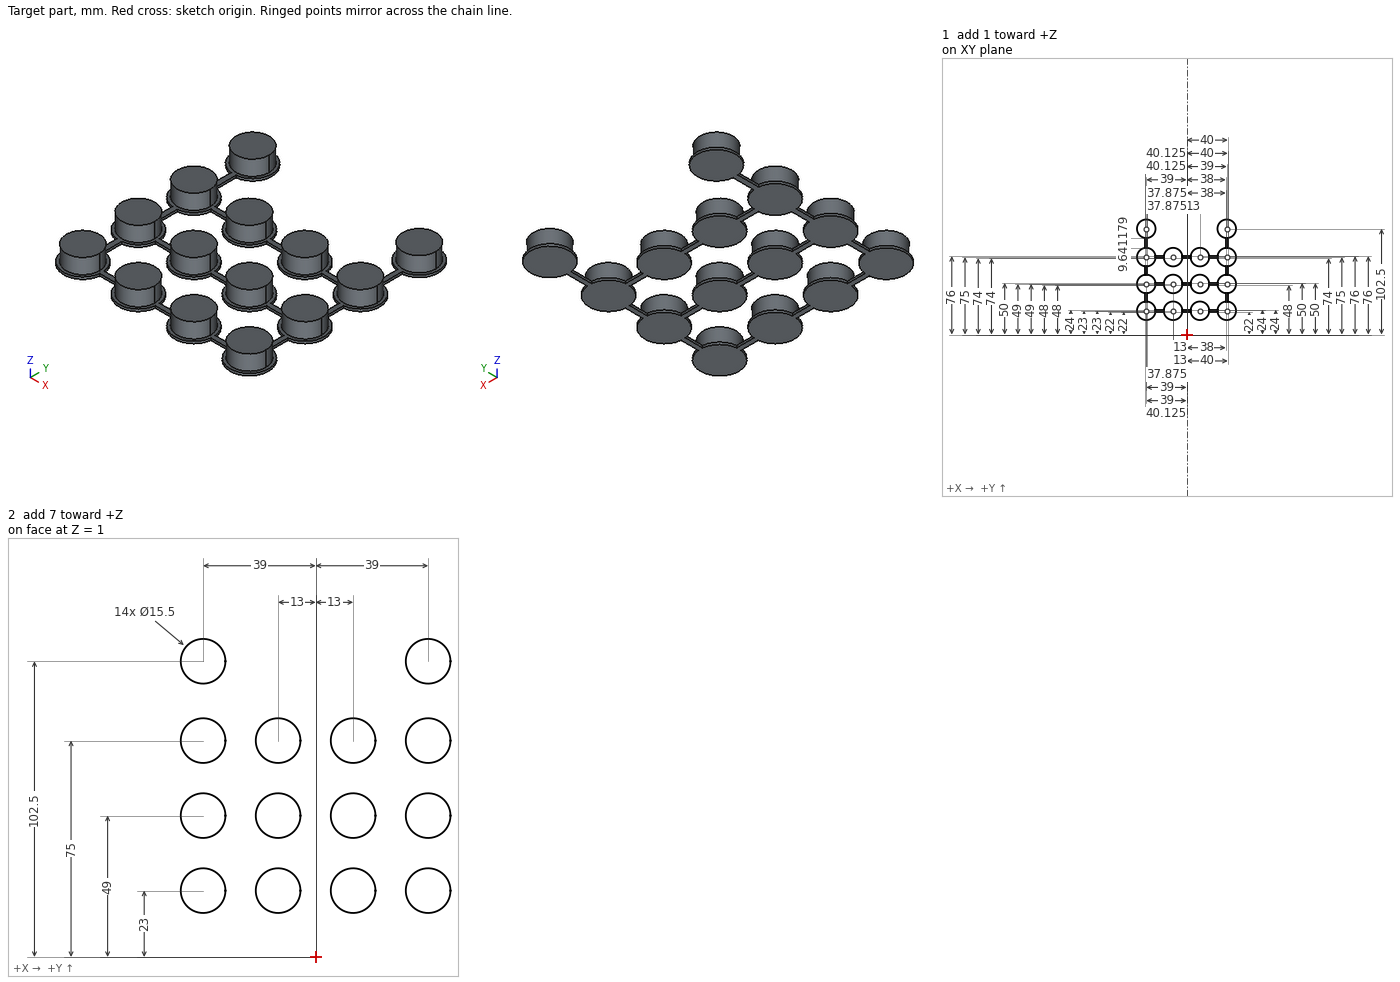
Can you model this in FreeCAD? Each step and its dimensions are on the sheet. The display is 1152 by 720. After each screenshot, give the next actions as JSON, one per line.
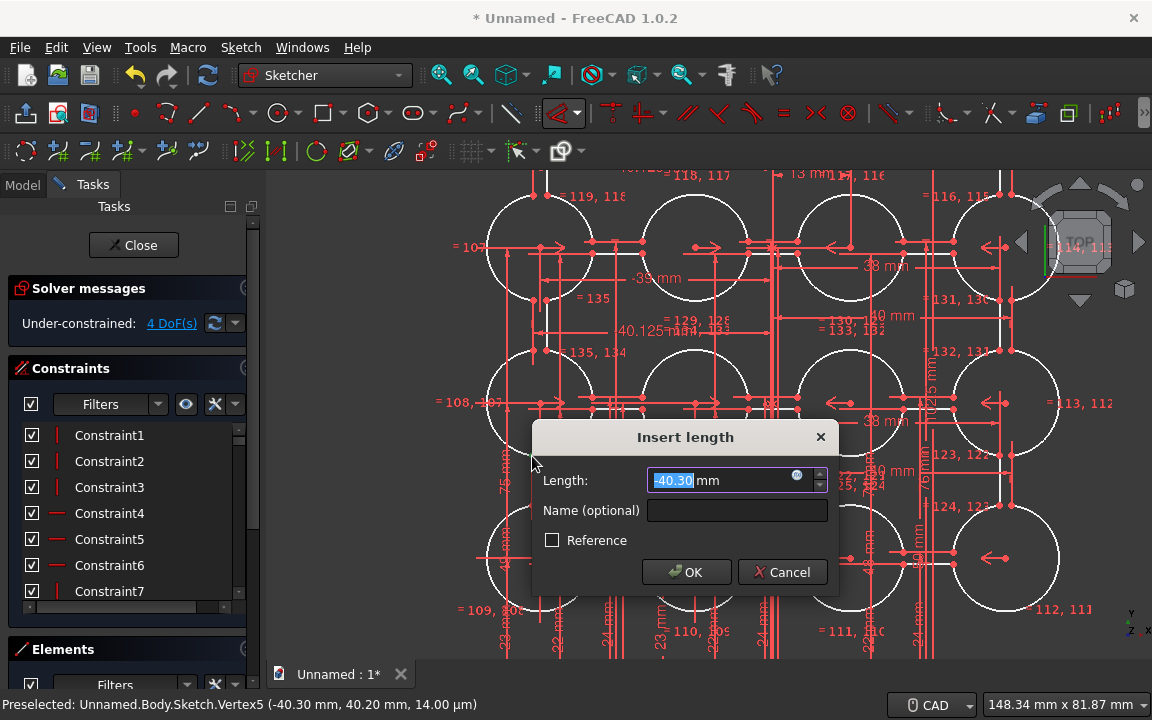
{"action": "type", "text": "-40.125"}
{"action": "key", "text": "Return"}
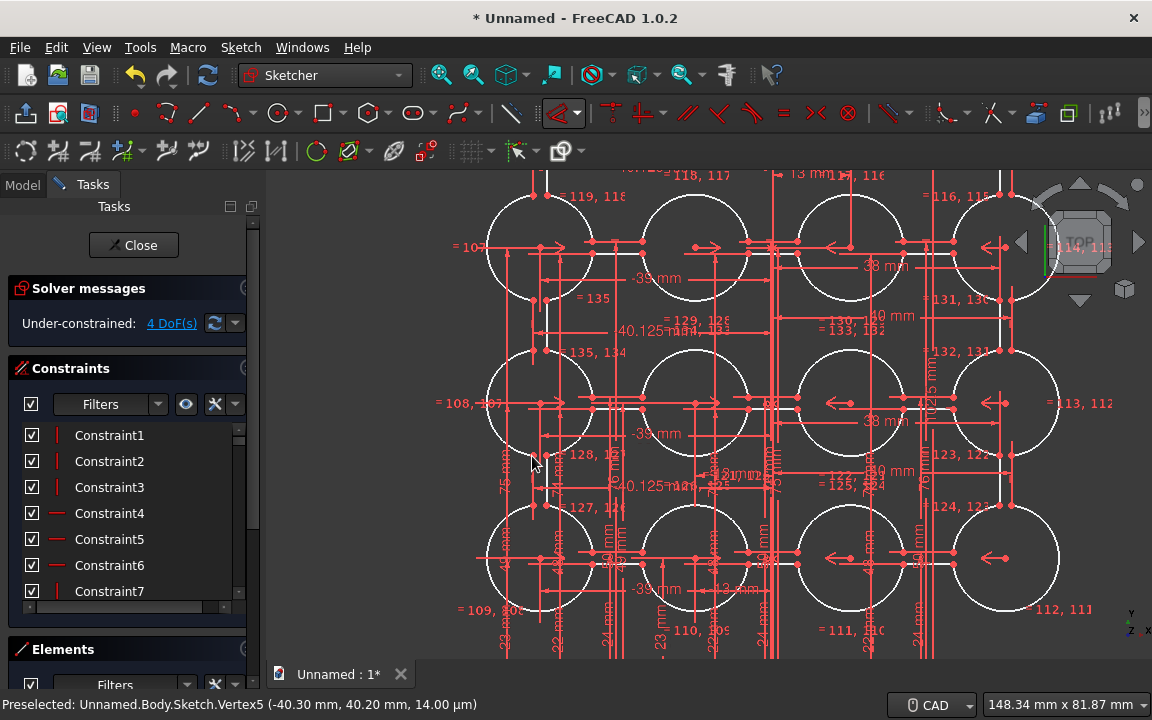
{"action": "scroll", "coordinate": [532, 457], "scroll_direction": "down", "scroll_amount": 4}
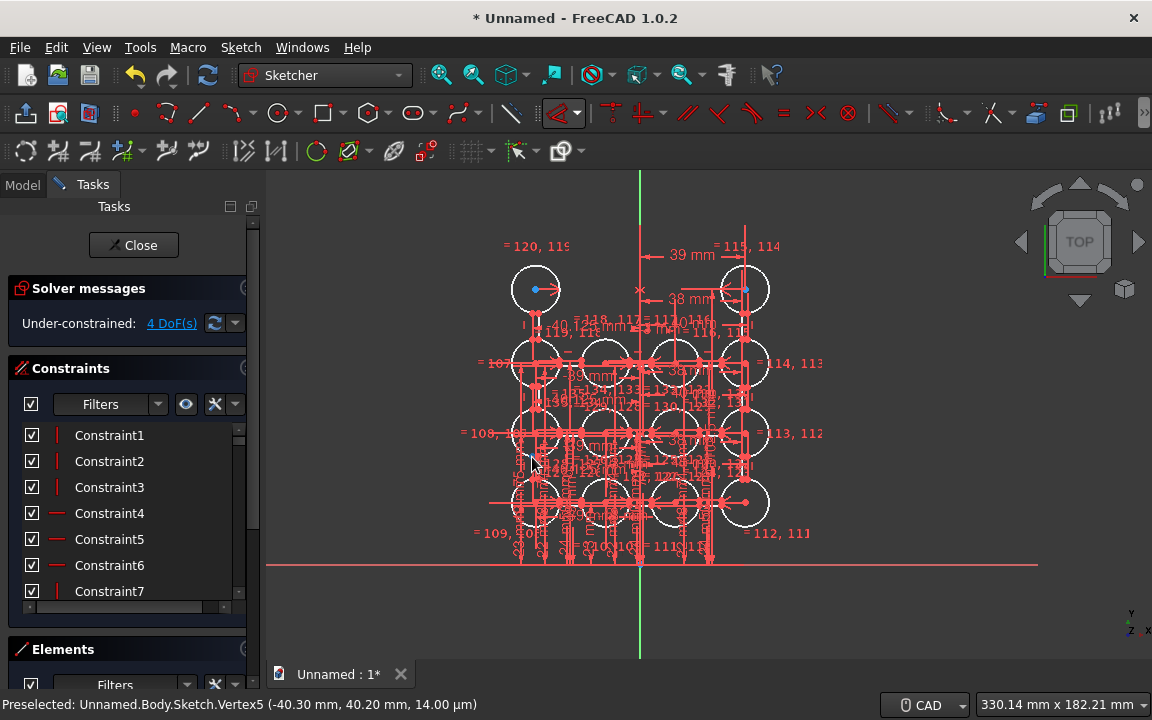
{"action": "scroll", "coordinate": [539, 340], "scroll_direction": "up", "scroll_amount": 4}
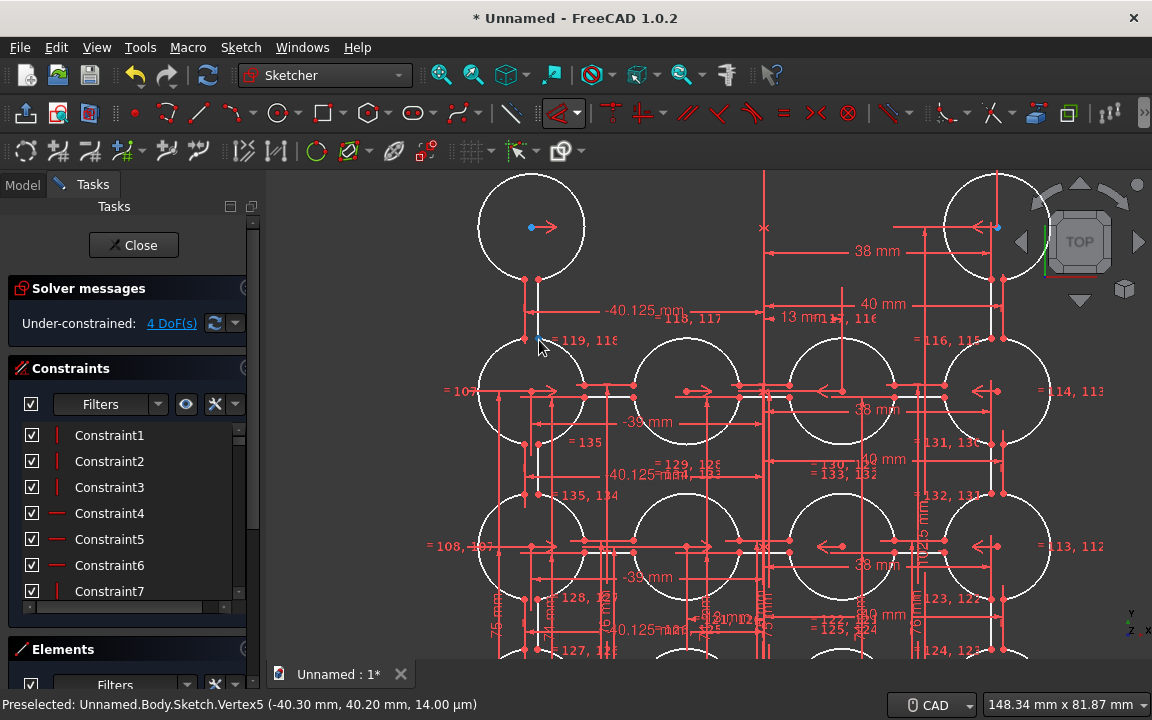
{"action": "left_click", "coordinate": [538, 339]}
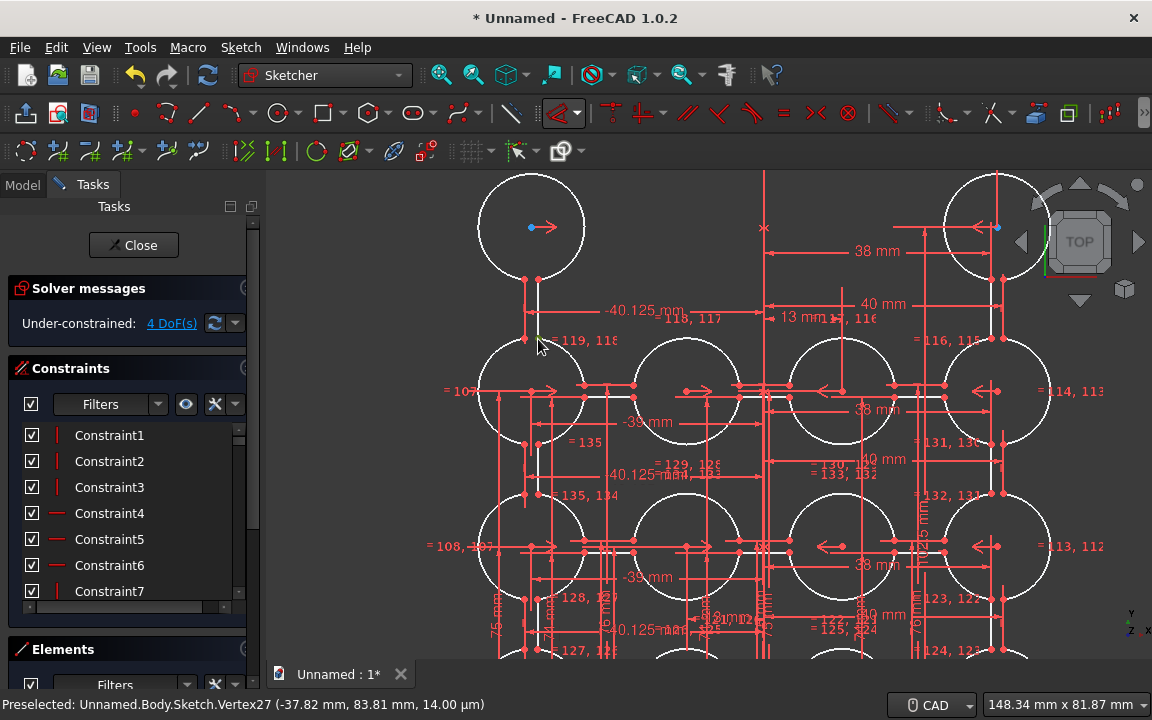
{"action": "left_click", "coordinate": [580, 114]}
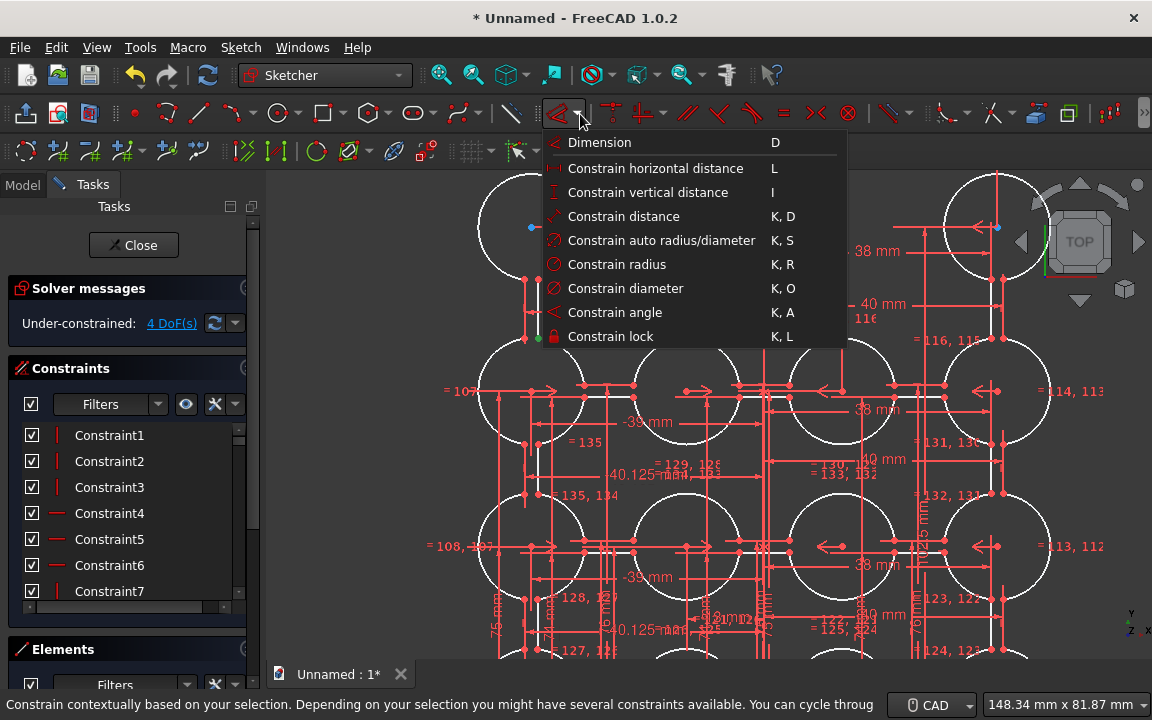
{"action": "left_click", "coordinate": [695, 168]}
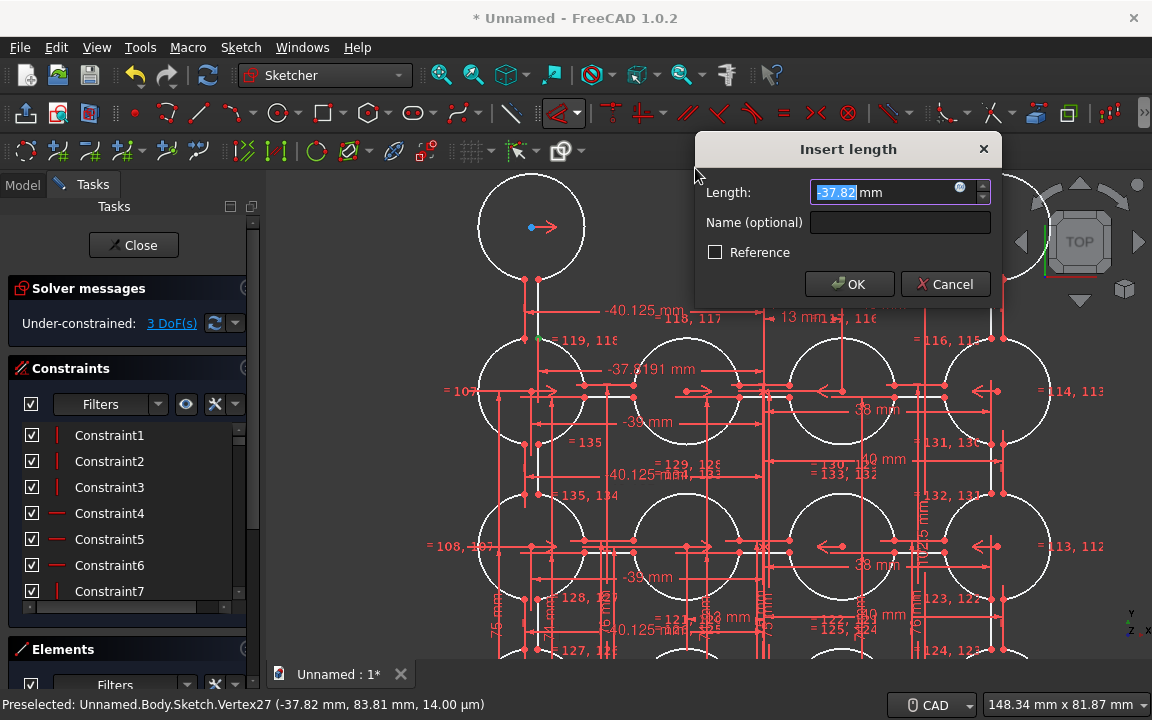
{"action": "type", "text": "-37.875"}
{"action": "key", "text": "Return"}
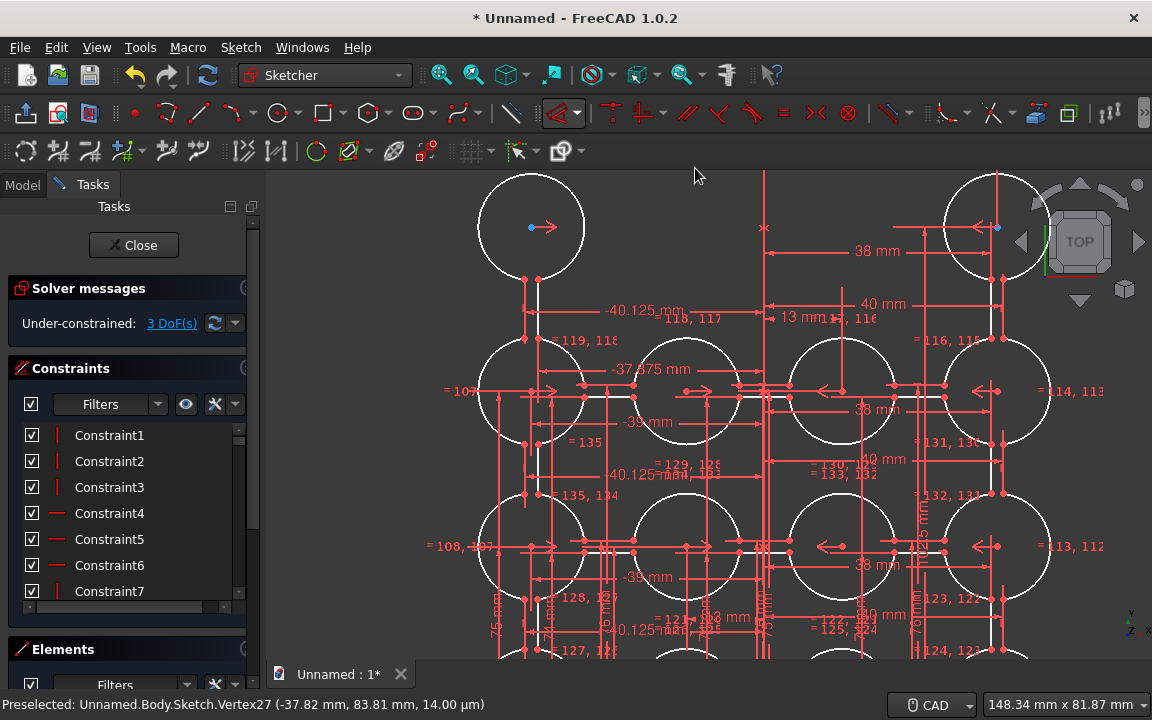
{"action": "scroll", "coordinate": [539, 340], "scroll_direction": "down", "scroll_amount": 4}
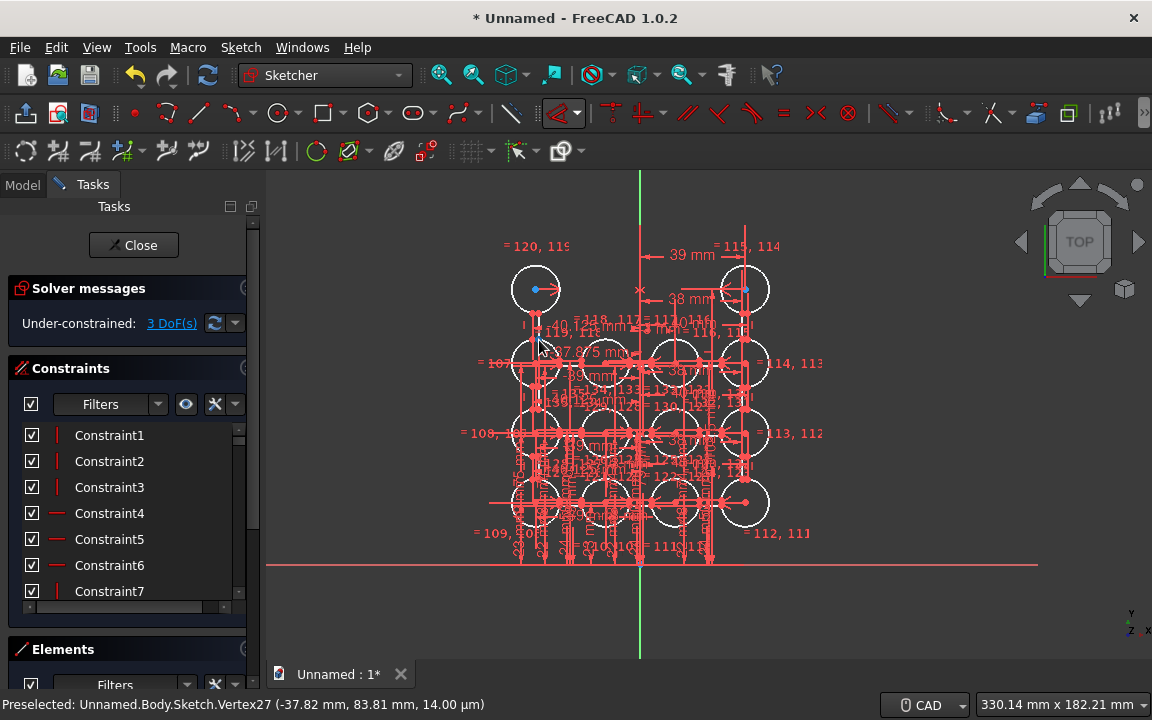
{"action": "scroll", "coordinate": [539, 479], "scroll_direction": "up", "scroll_amount": 4}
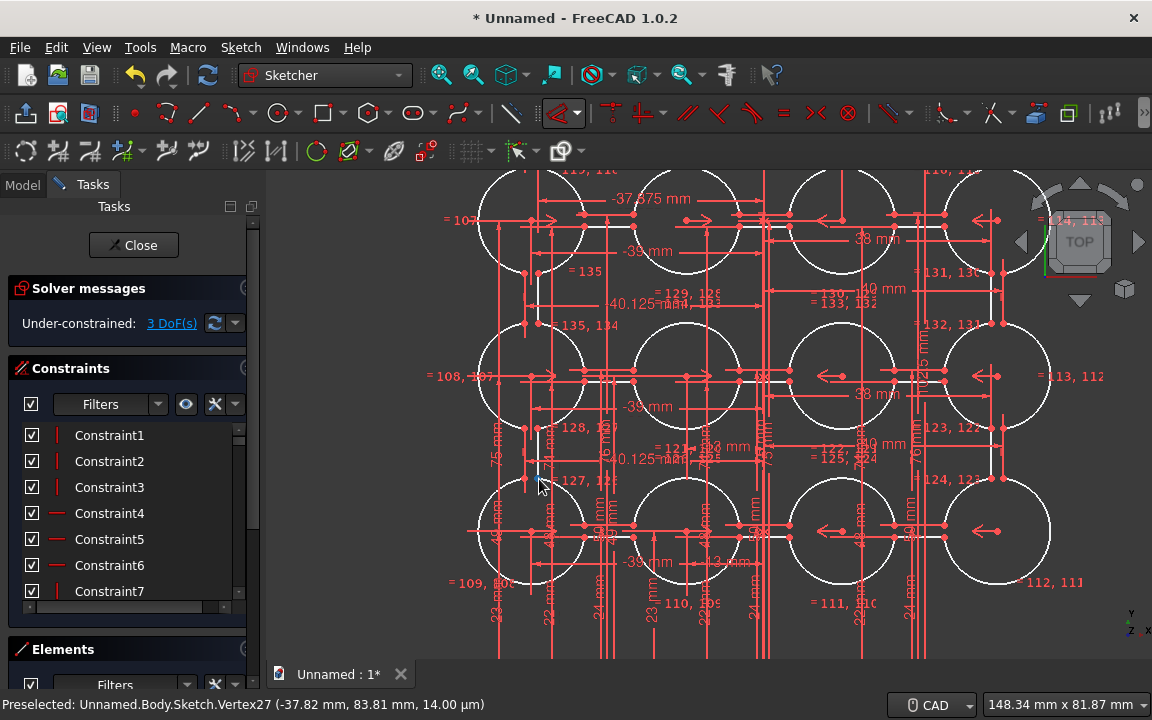
{"action": "left_click", "coordinate": [538, 479]}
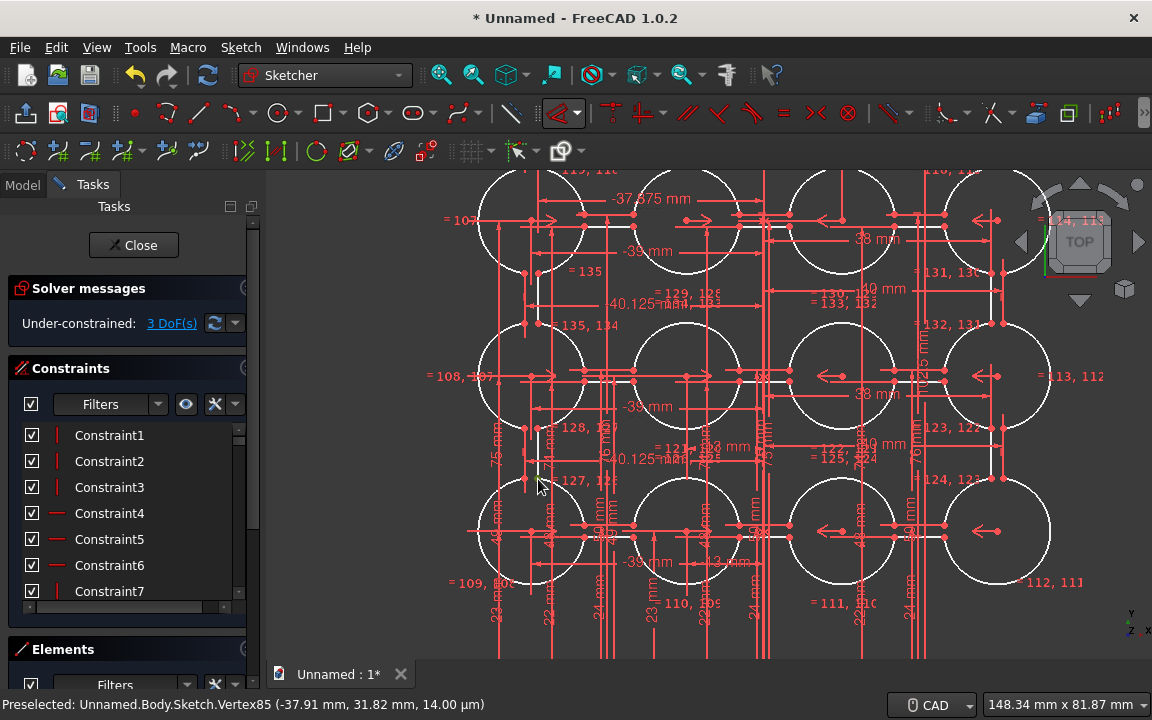
{"action": "left_click", "coordinate": [580, 114]}